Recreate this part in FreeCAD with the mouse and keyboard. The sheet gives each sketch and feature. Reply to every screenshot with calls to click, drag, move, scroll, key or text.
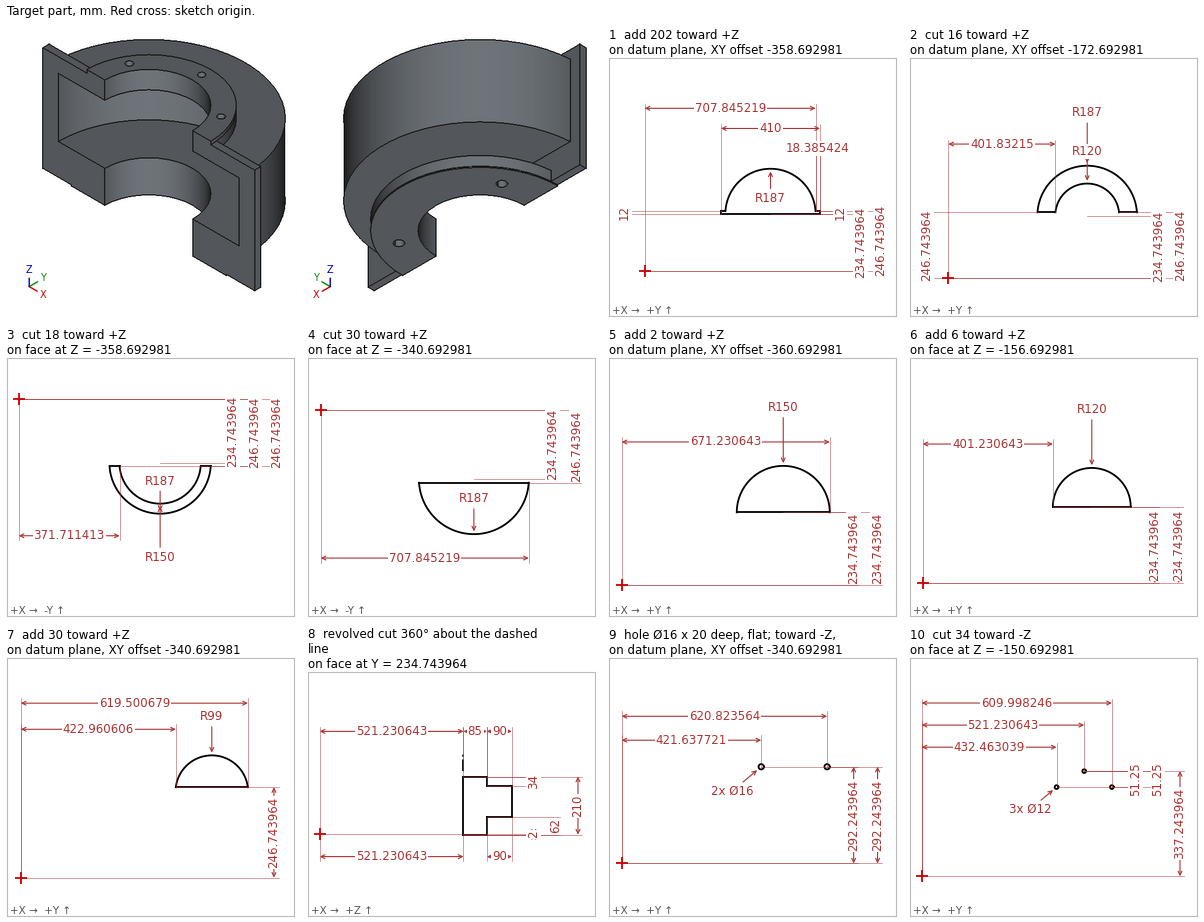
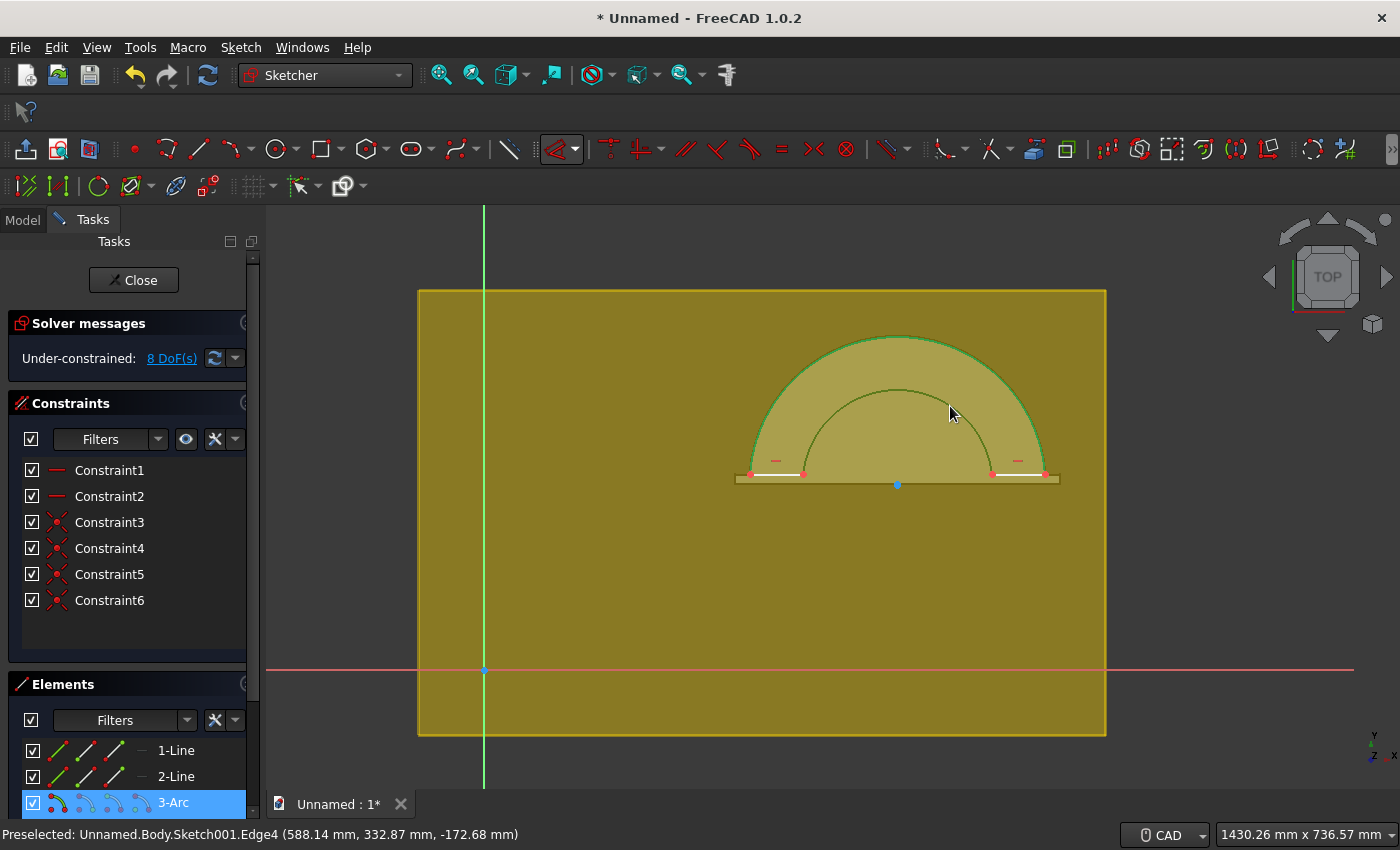
click(610, 150)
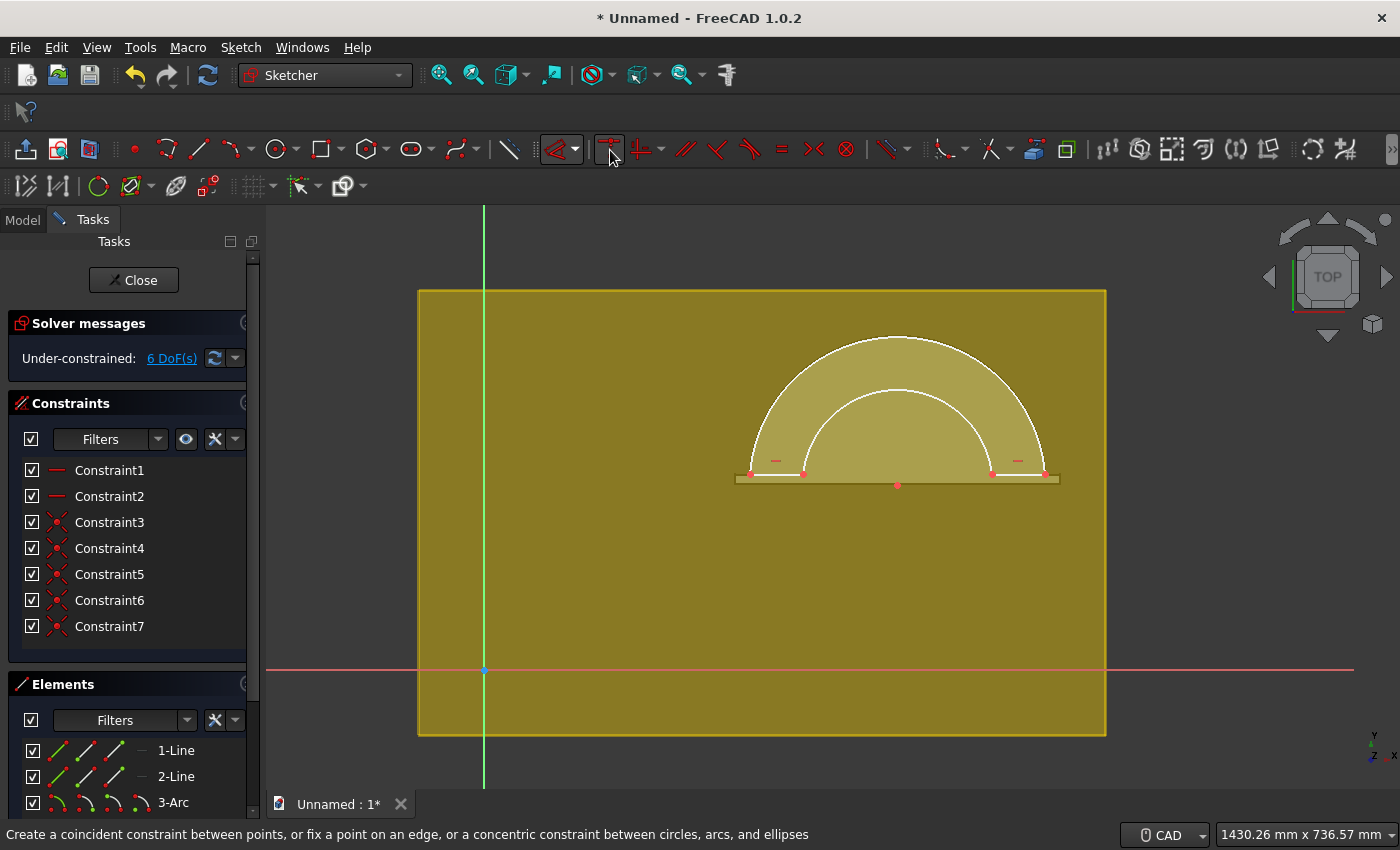
key(d)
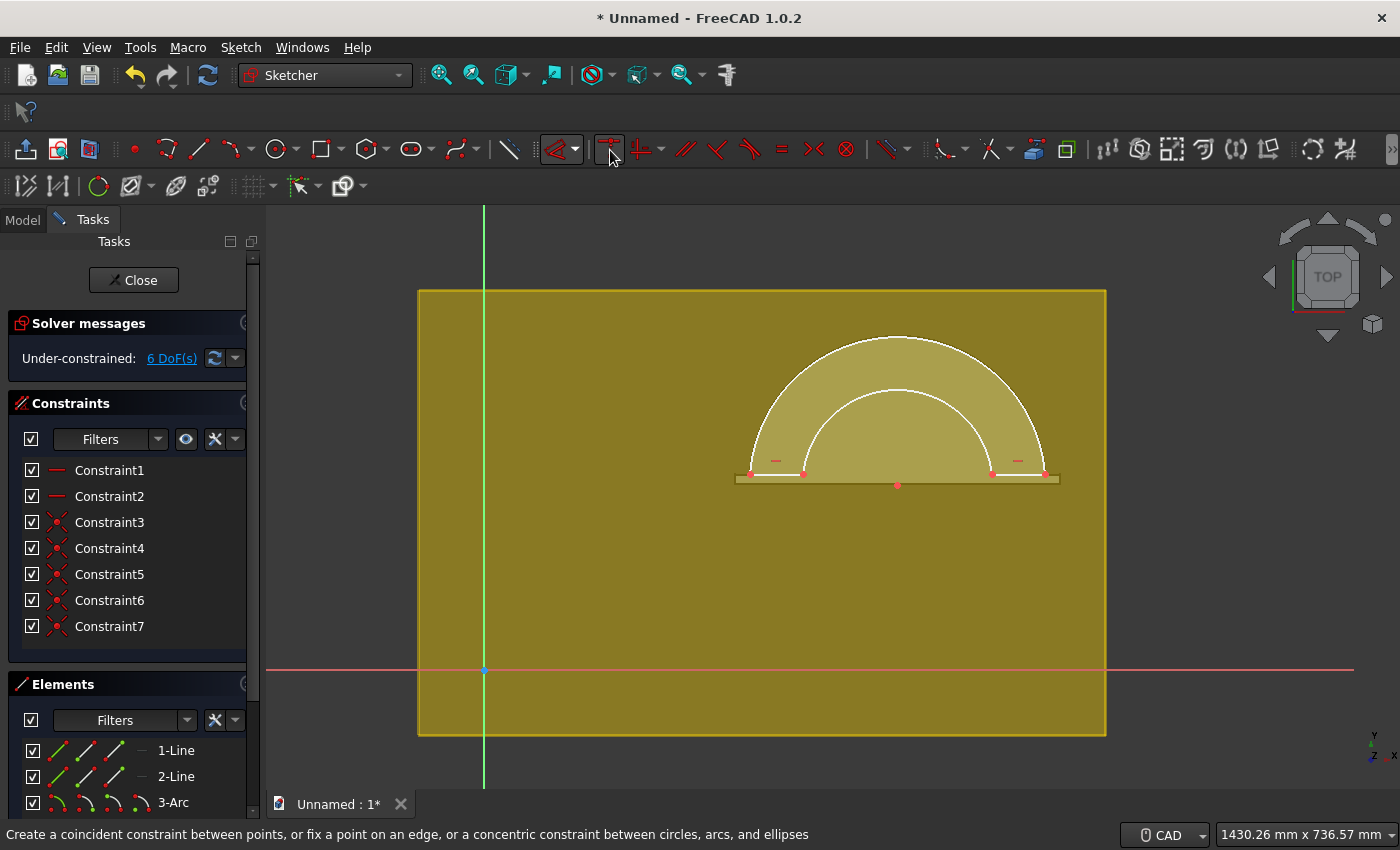
click(981, 363)
click(999, 337)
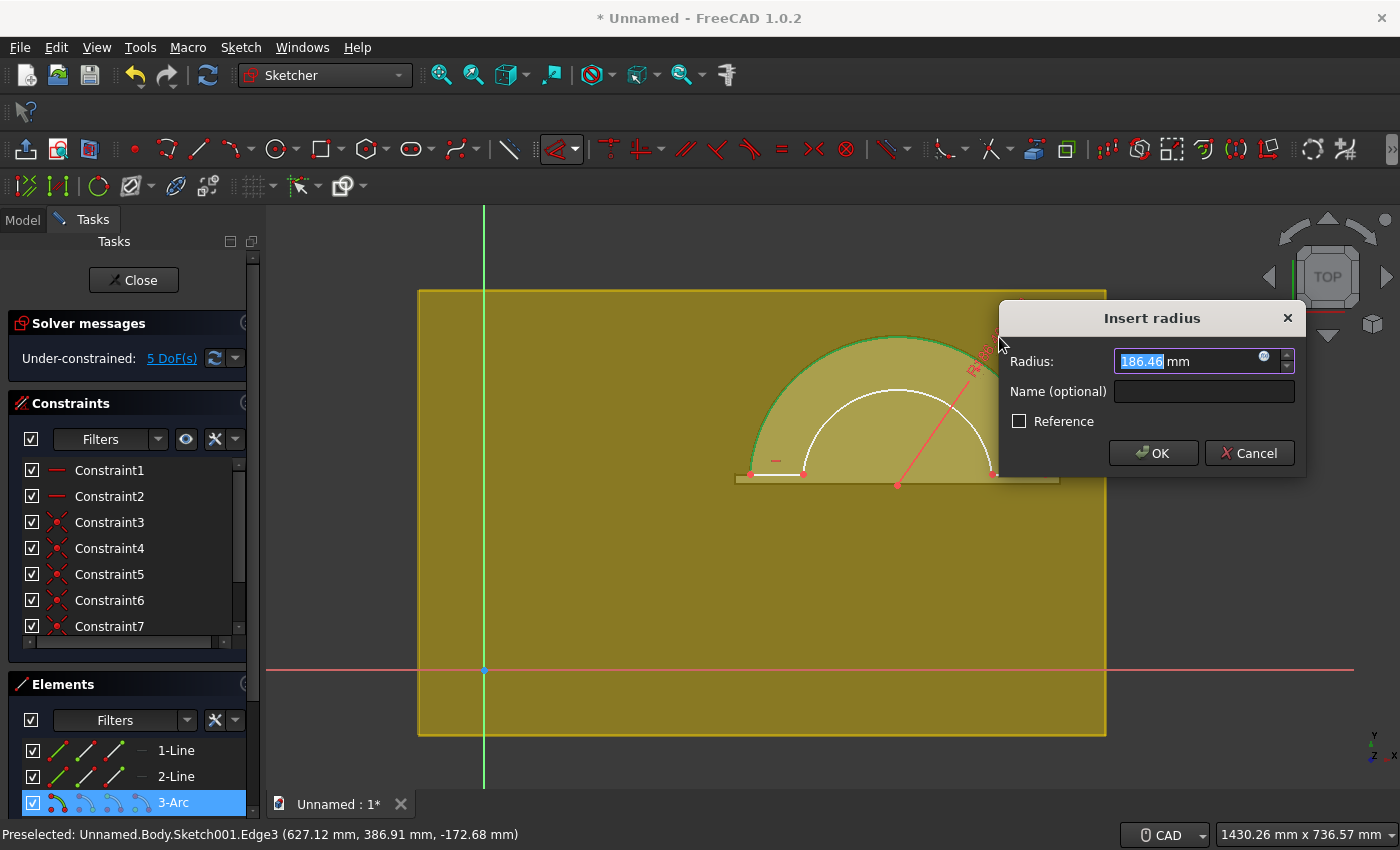
text(187)
key(Return)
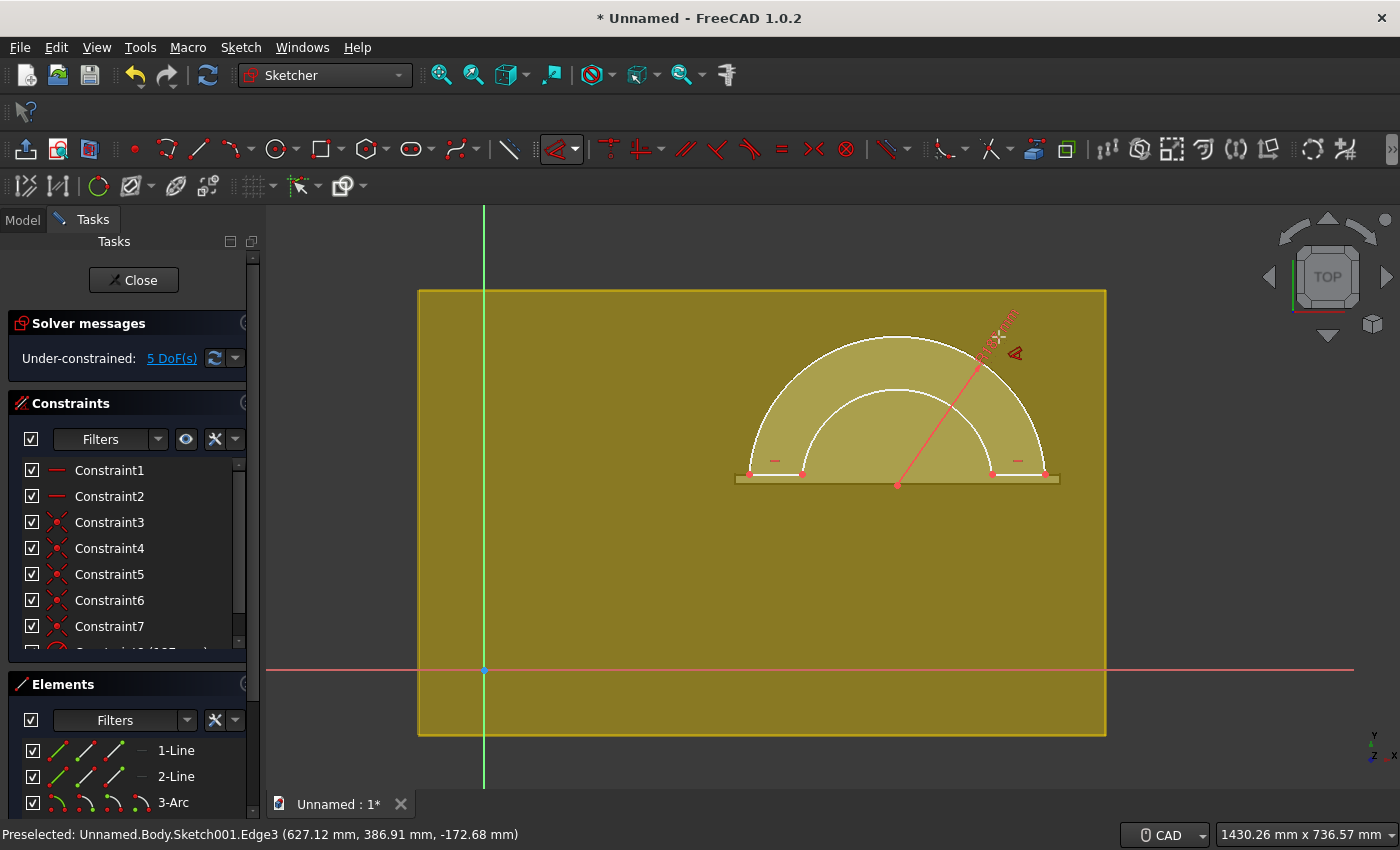
click(950, 406)
click(968, 379)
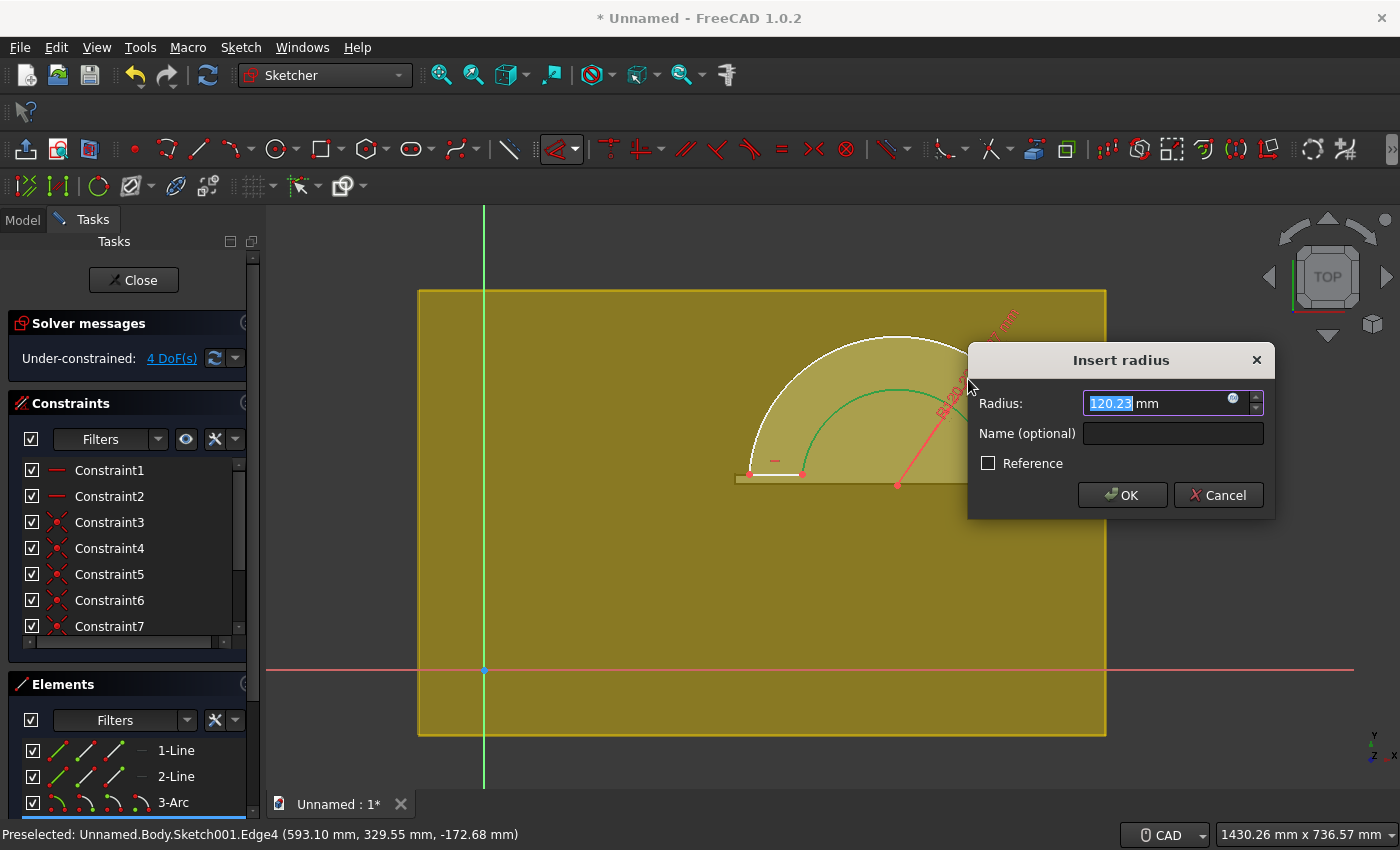
text(120)
key(Return)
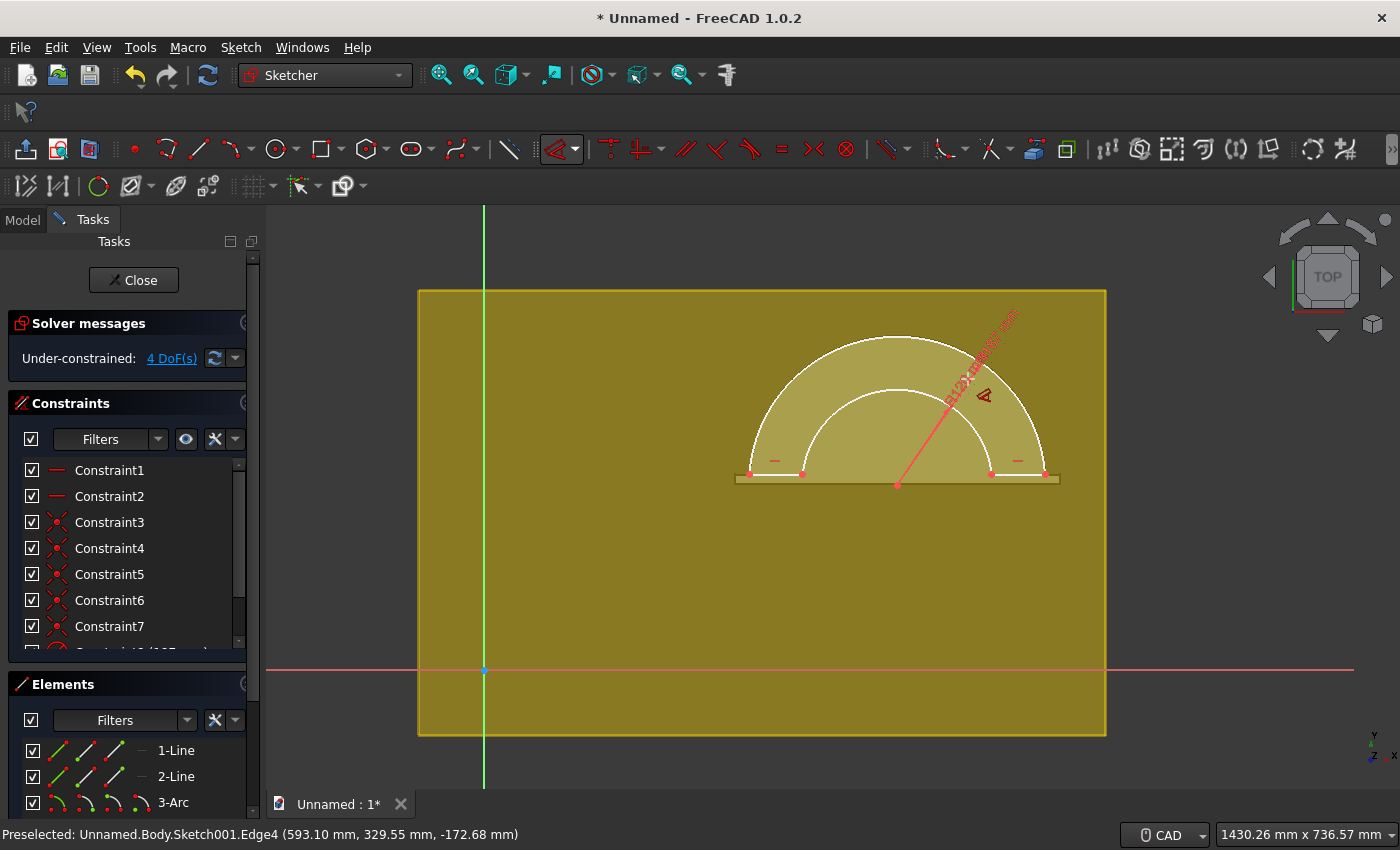
click(803, 475)
click(643, 704)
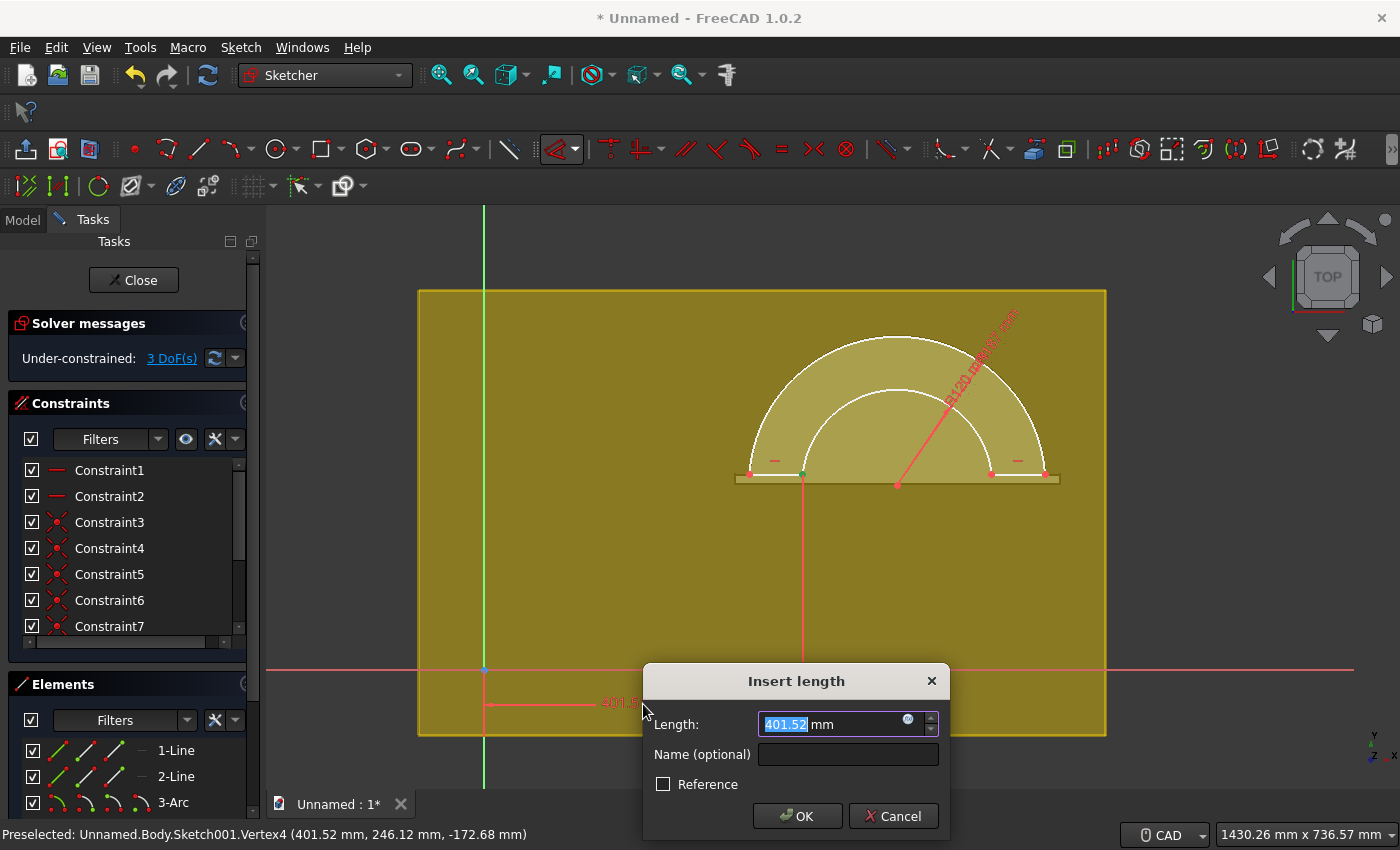
text(401.83215)
key(Return)